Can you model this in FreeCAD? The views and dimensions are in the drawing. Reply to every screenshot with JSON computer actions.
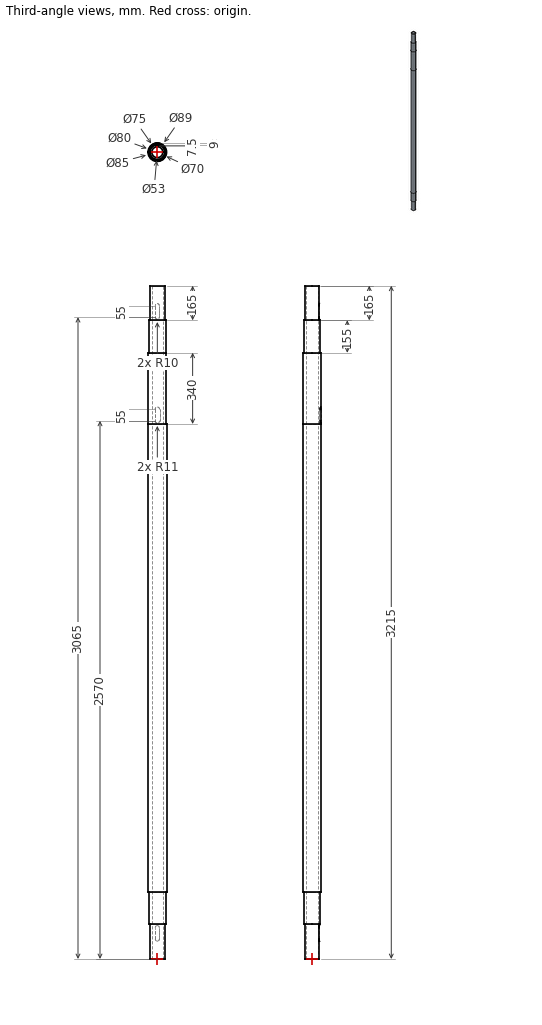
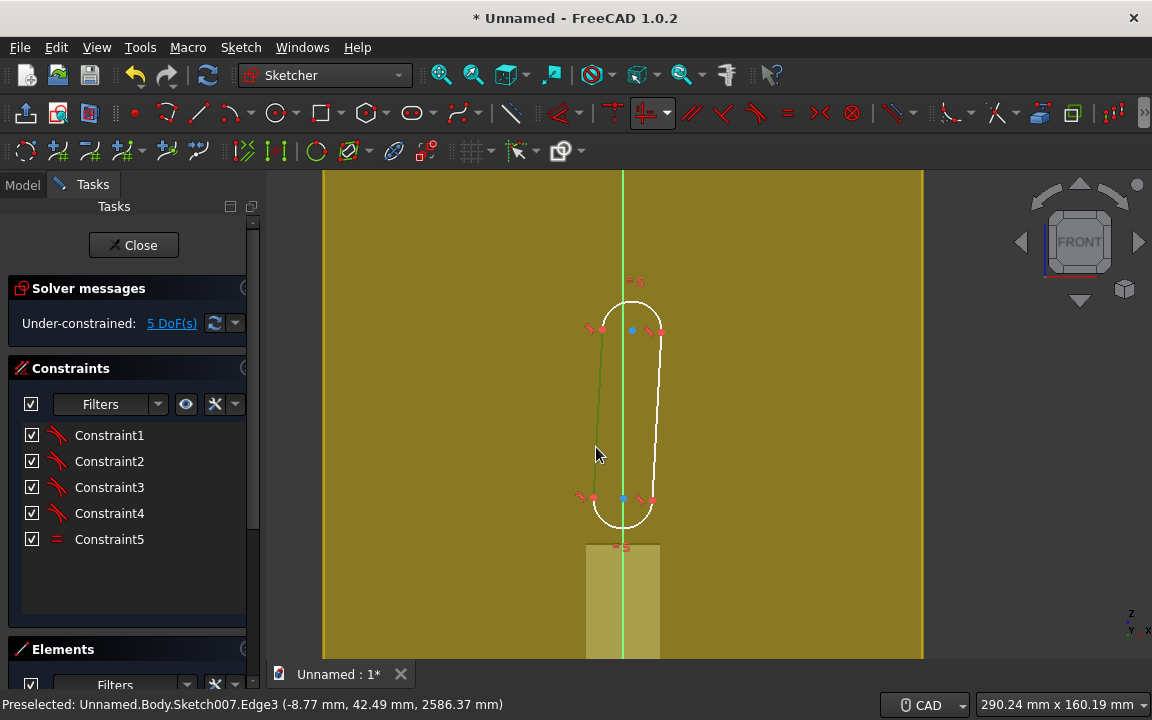
{"action": "left_click", "coordinate": [670, 114]}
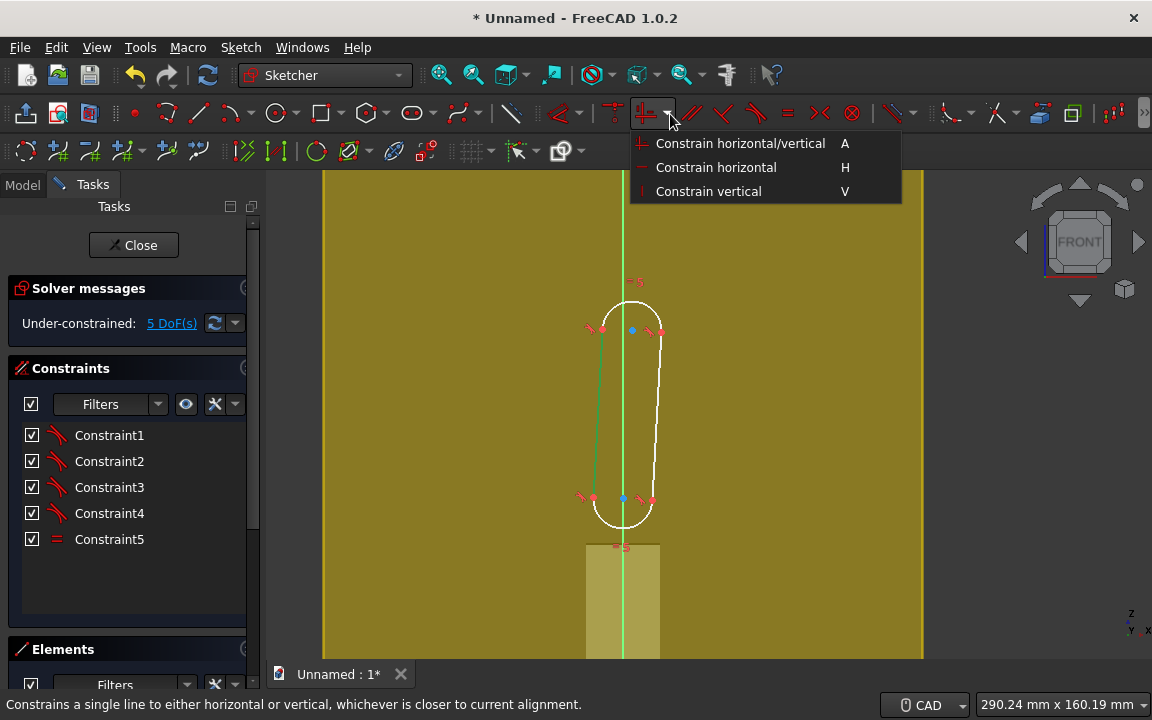
{"action": "left_click", "coordinate": [766, 191]}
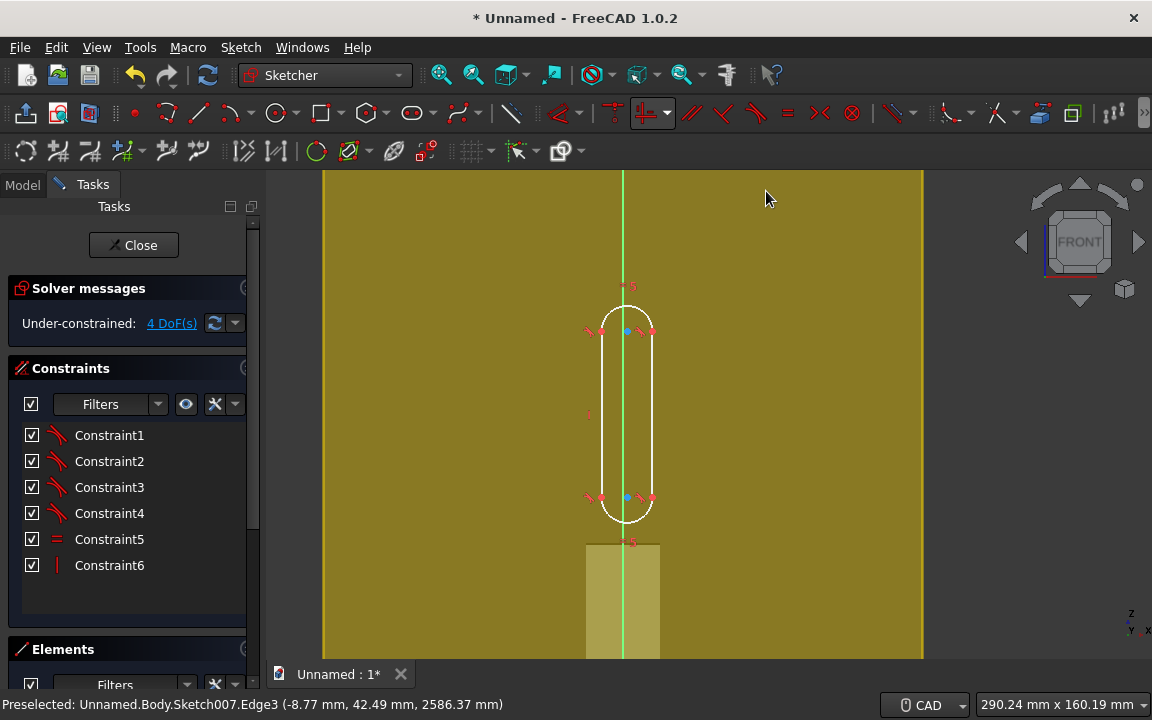
{"action": "left_click", "coordinate": [627, 497]}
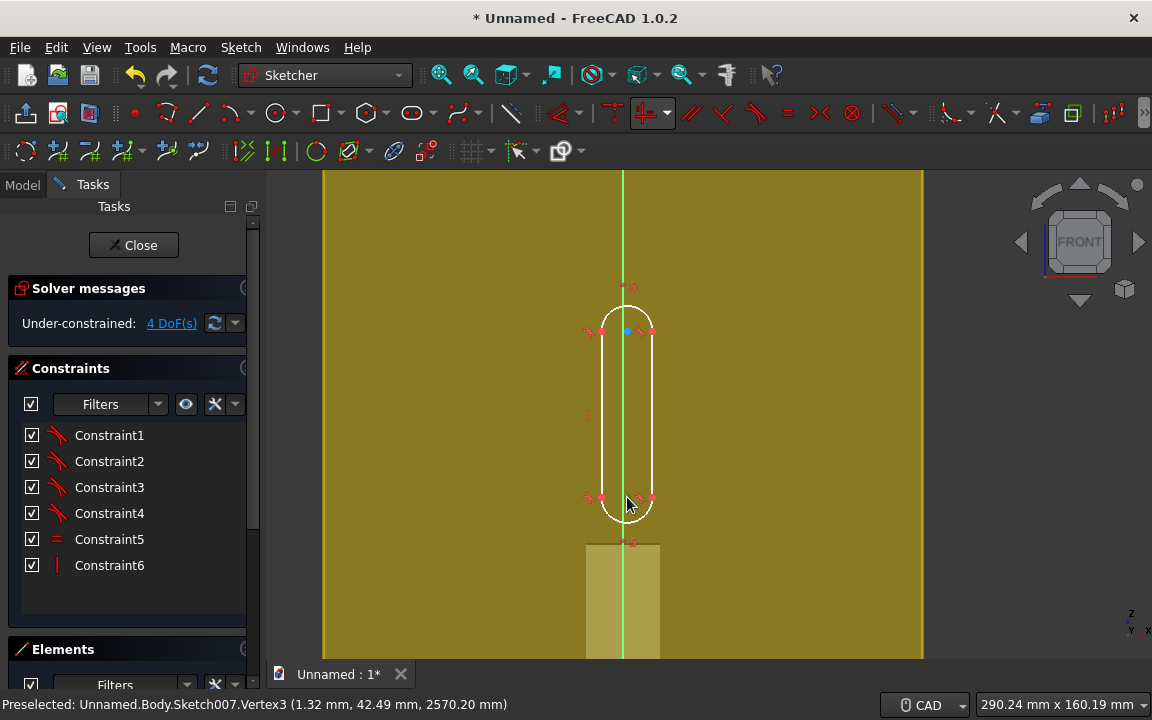
{"action": "left_click", "coordinate": [623, 600]}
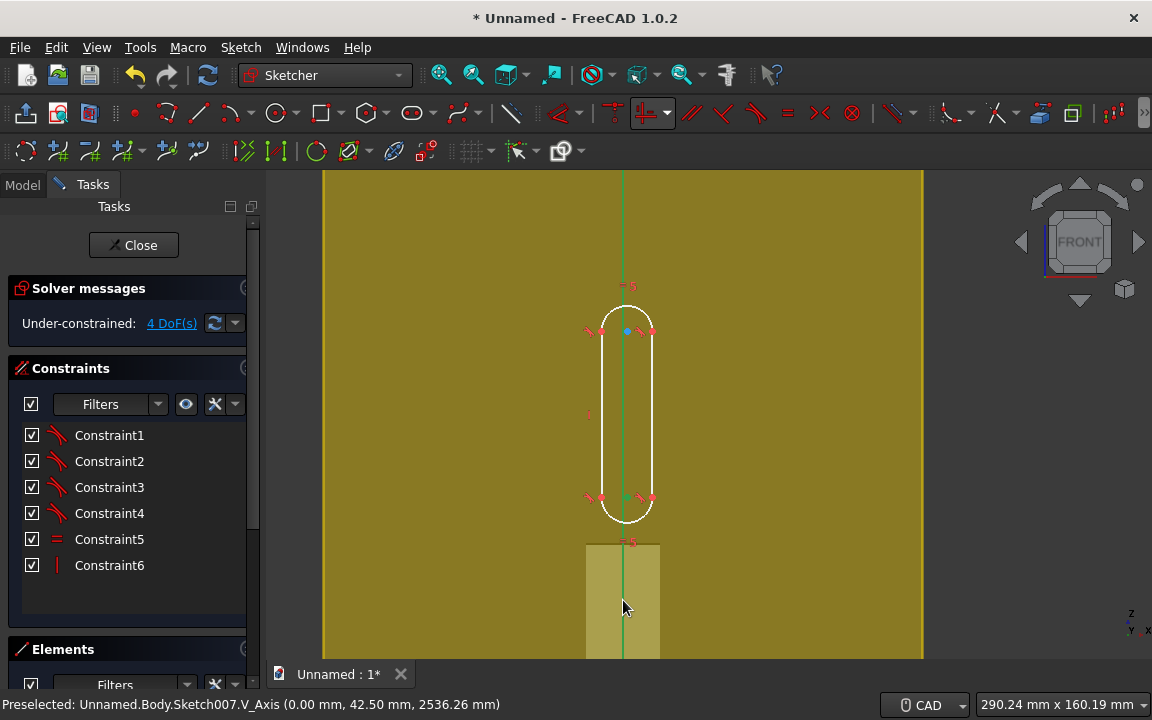
{"action": "left_click", "coordinate": [614, 114]}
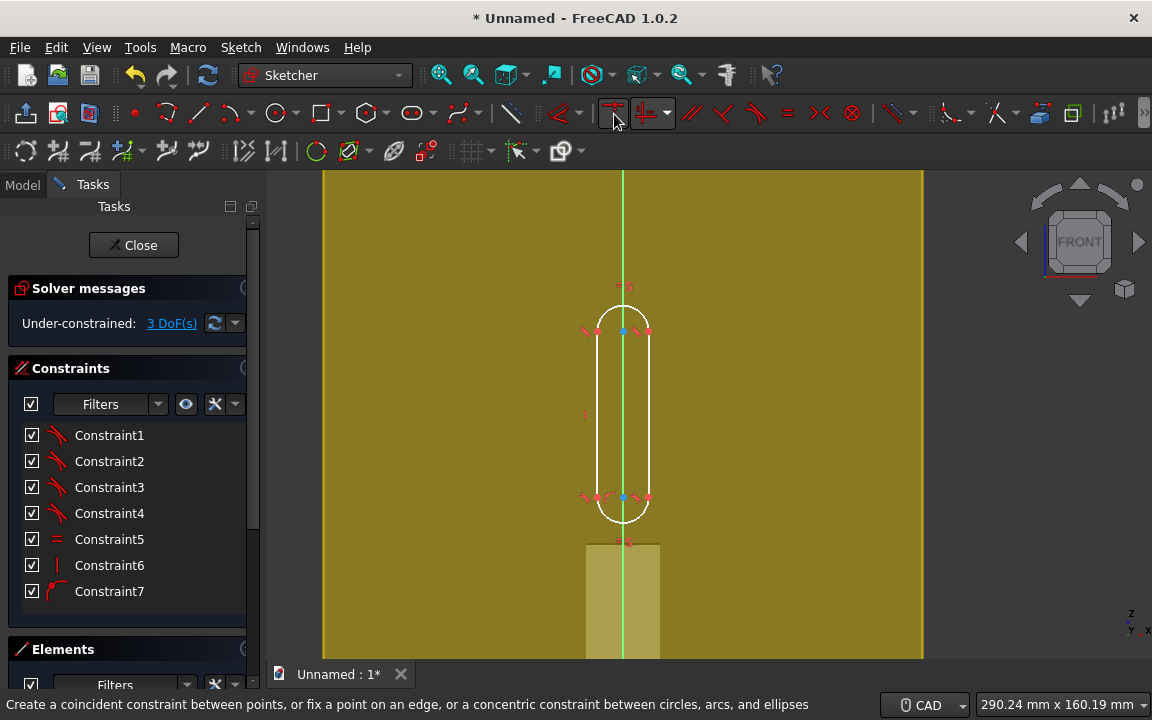
{"action": "left_click", "coordinate": [558, 114]}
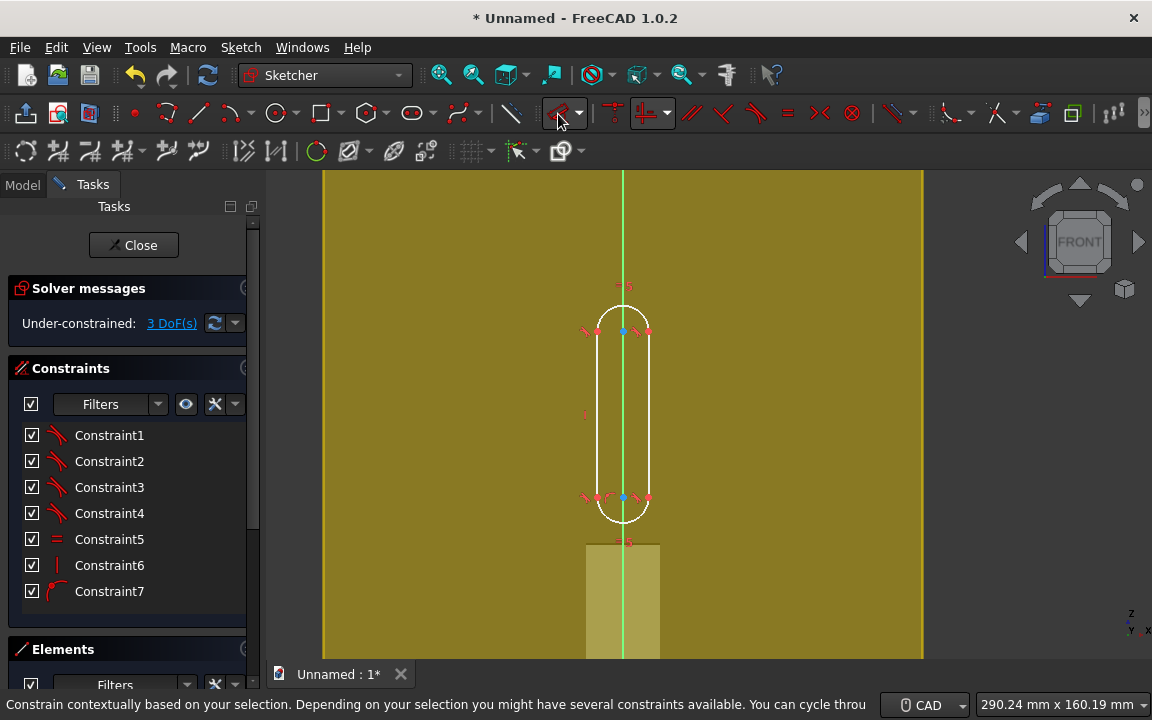
{"action": "left_click", "coordinate": [608, 518]}
{"action": "left_click", "coordinate": [589, 544]}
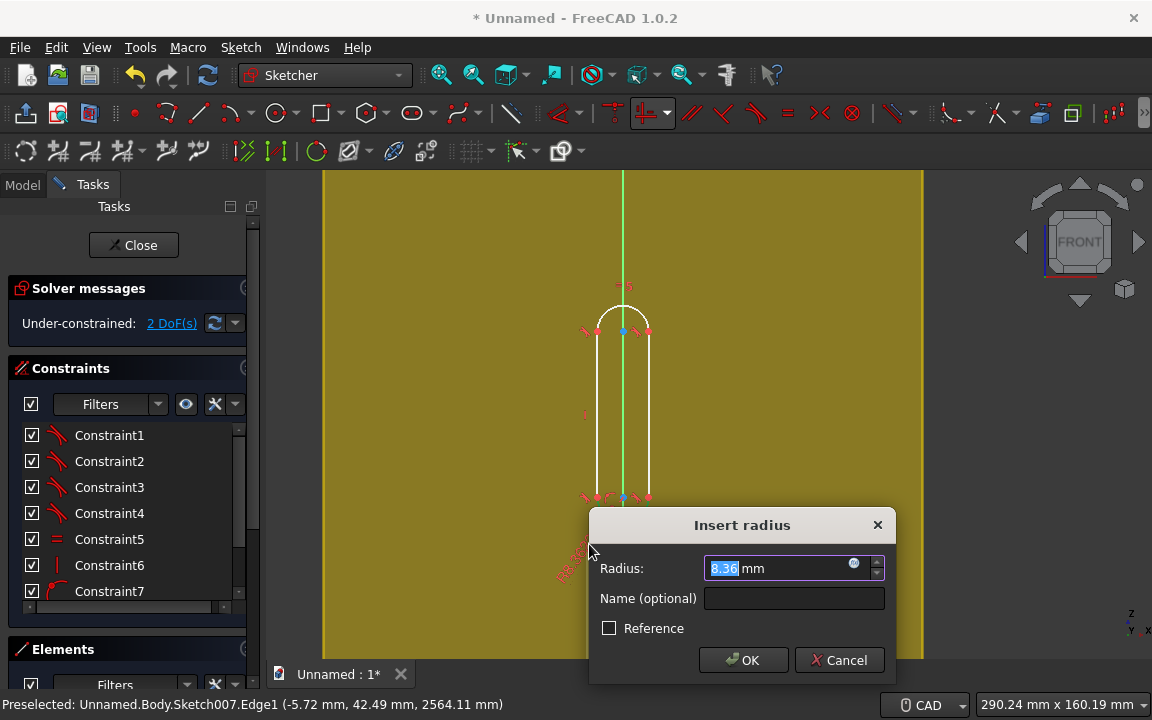
{"action": "type", "text": "11"}
{"action": "key", "text": "Return"}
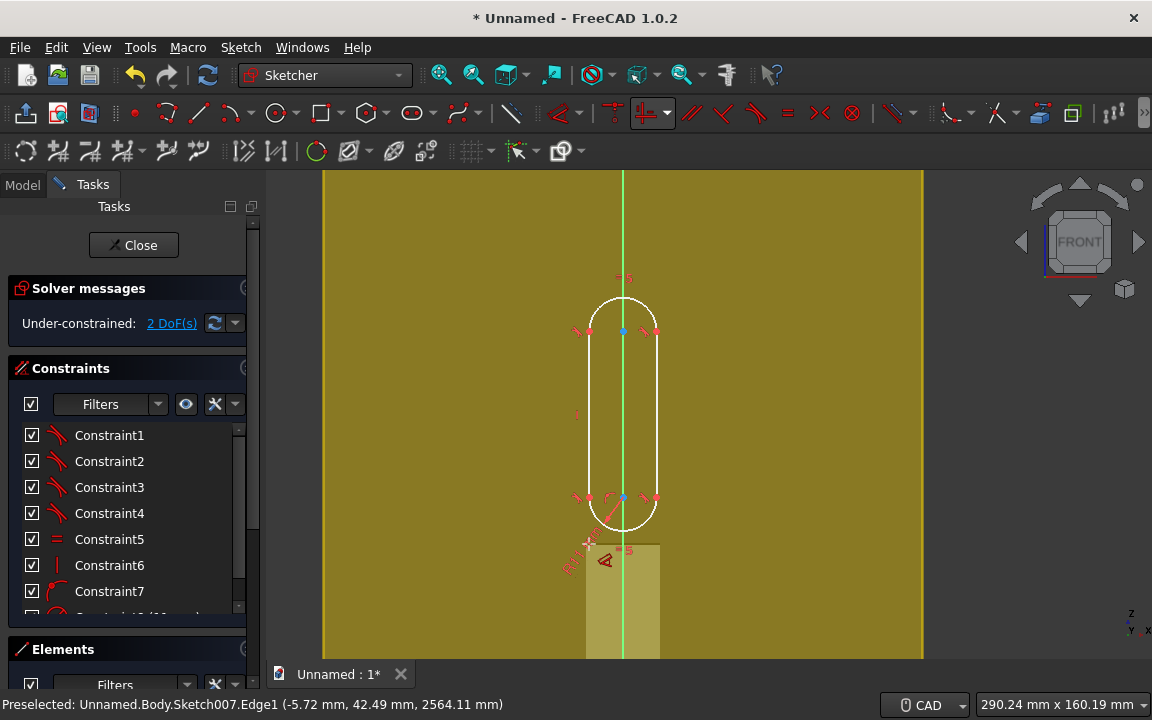
{"action": "left_click", "coordinate": [589, 448]}
{"action": "left_click", "coordinate": [555, 414]}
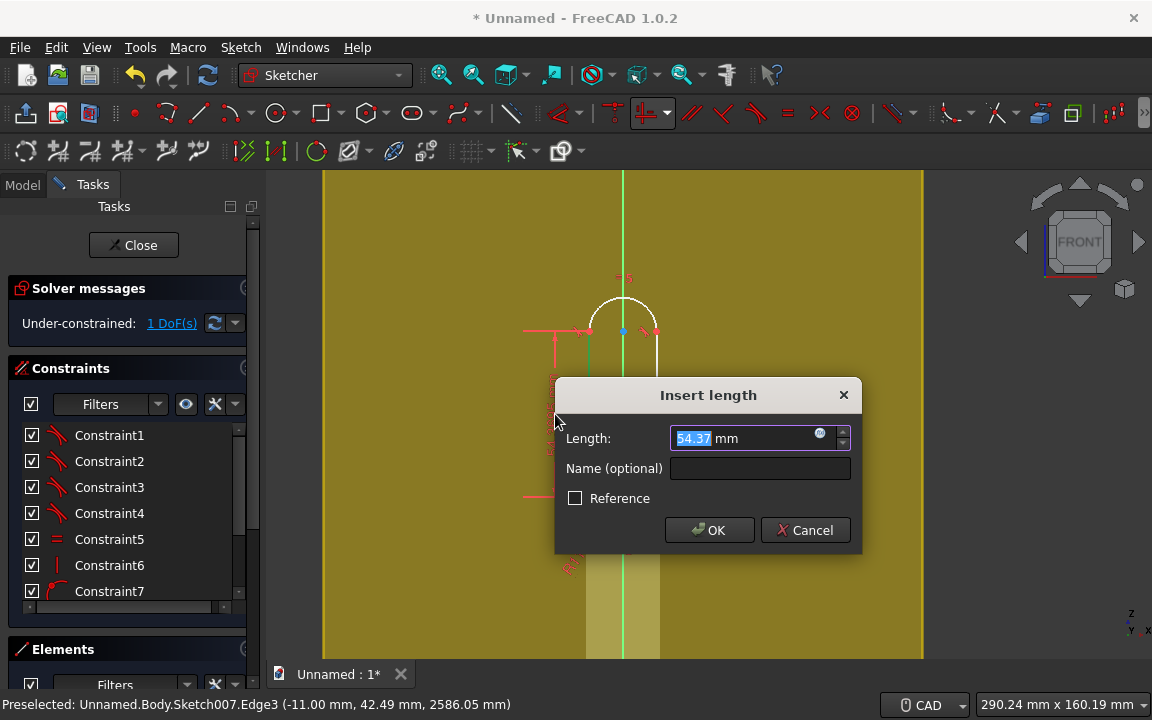
{"action": "type", "text": "55"}
{"action": "key", "text": "Return"}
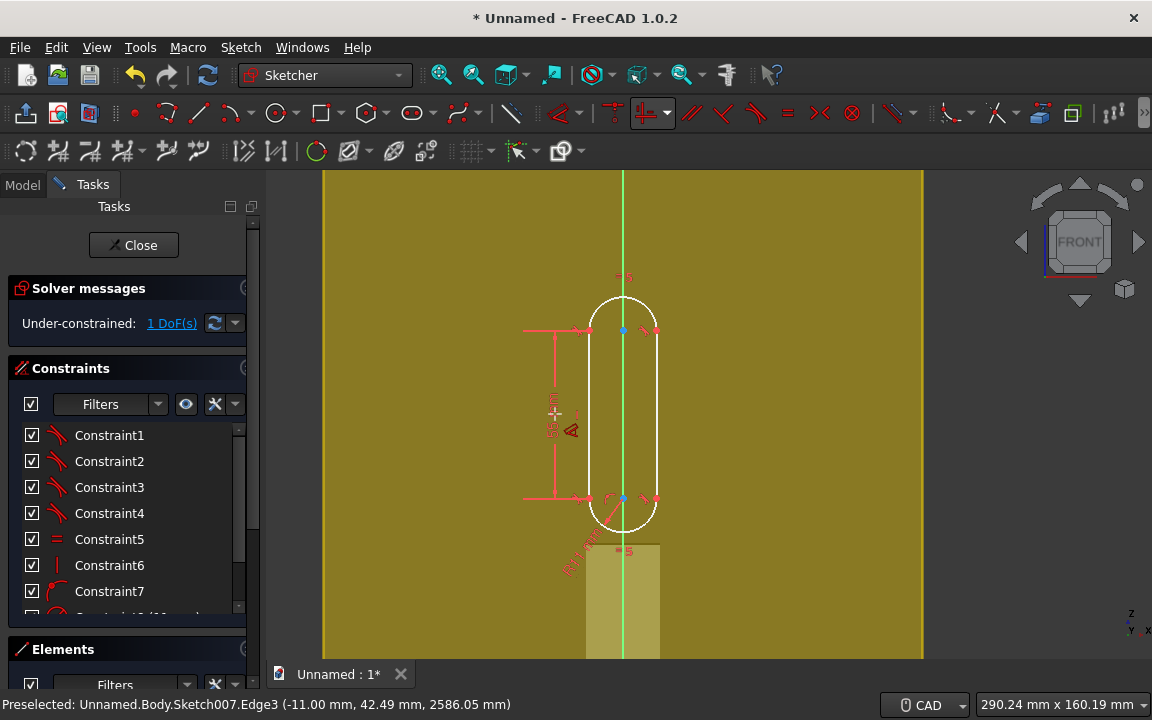
{"action": "left_click", "coordinate": [589, 499]}
{"action": "left_click", "coordinate": [555, 565]}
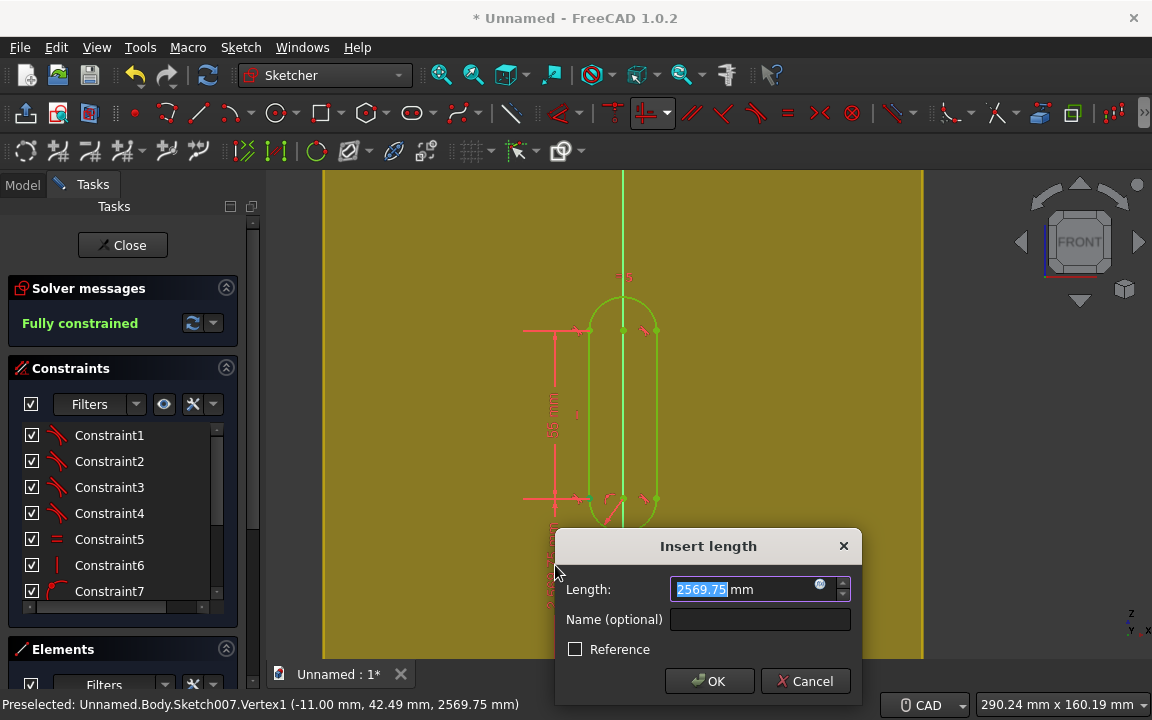
{"action": "type", "text": "2570"}
{"action": "key", "text": "Return"}
{"action": "key", "text": "Escape"}